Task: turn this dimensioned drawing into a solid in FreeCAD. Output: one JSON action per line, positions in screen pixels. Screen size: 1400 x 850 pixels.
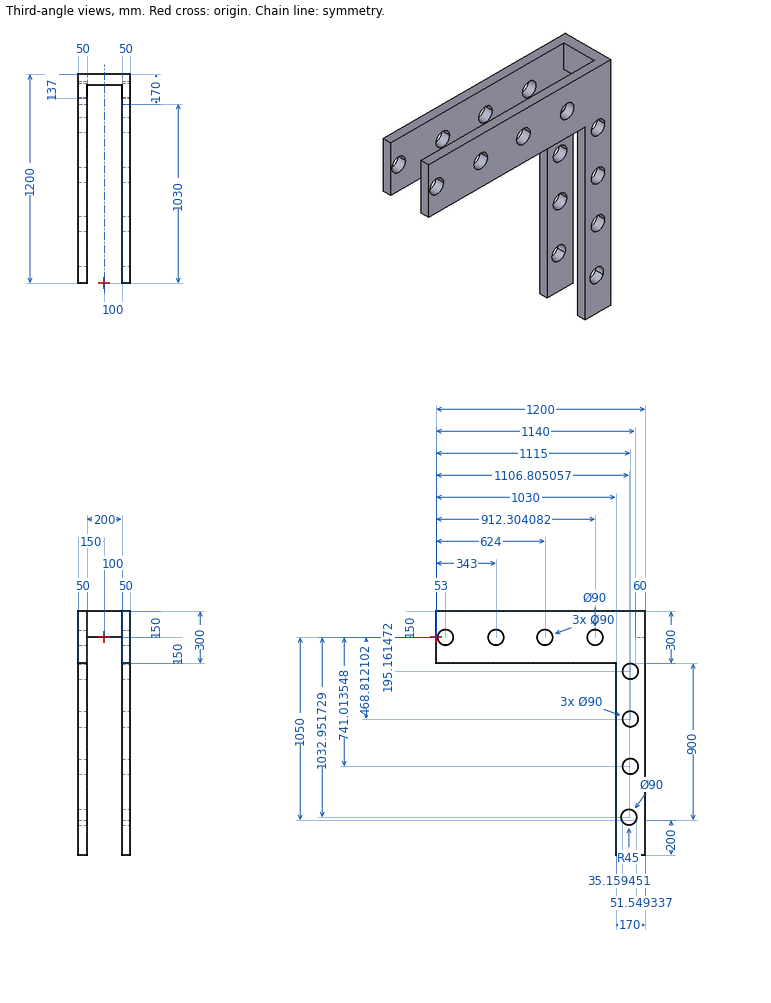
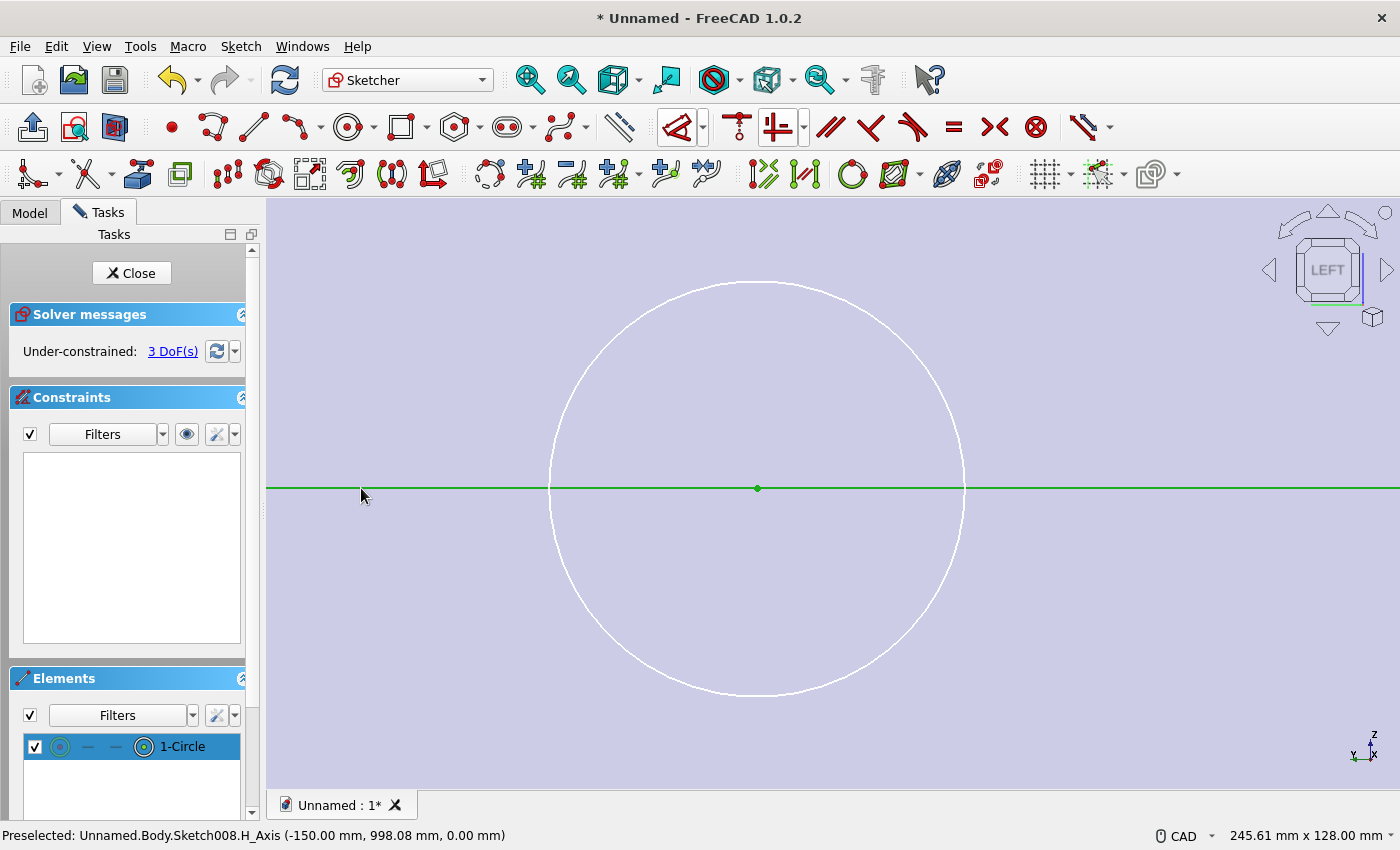
{"action": "left_click", "coordinate": [737, 128]}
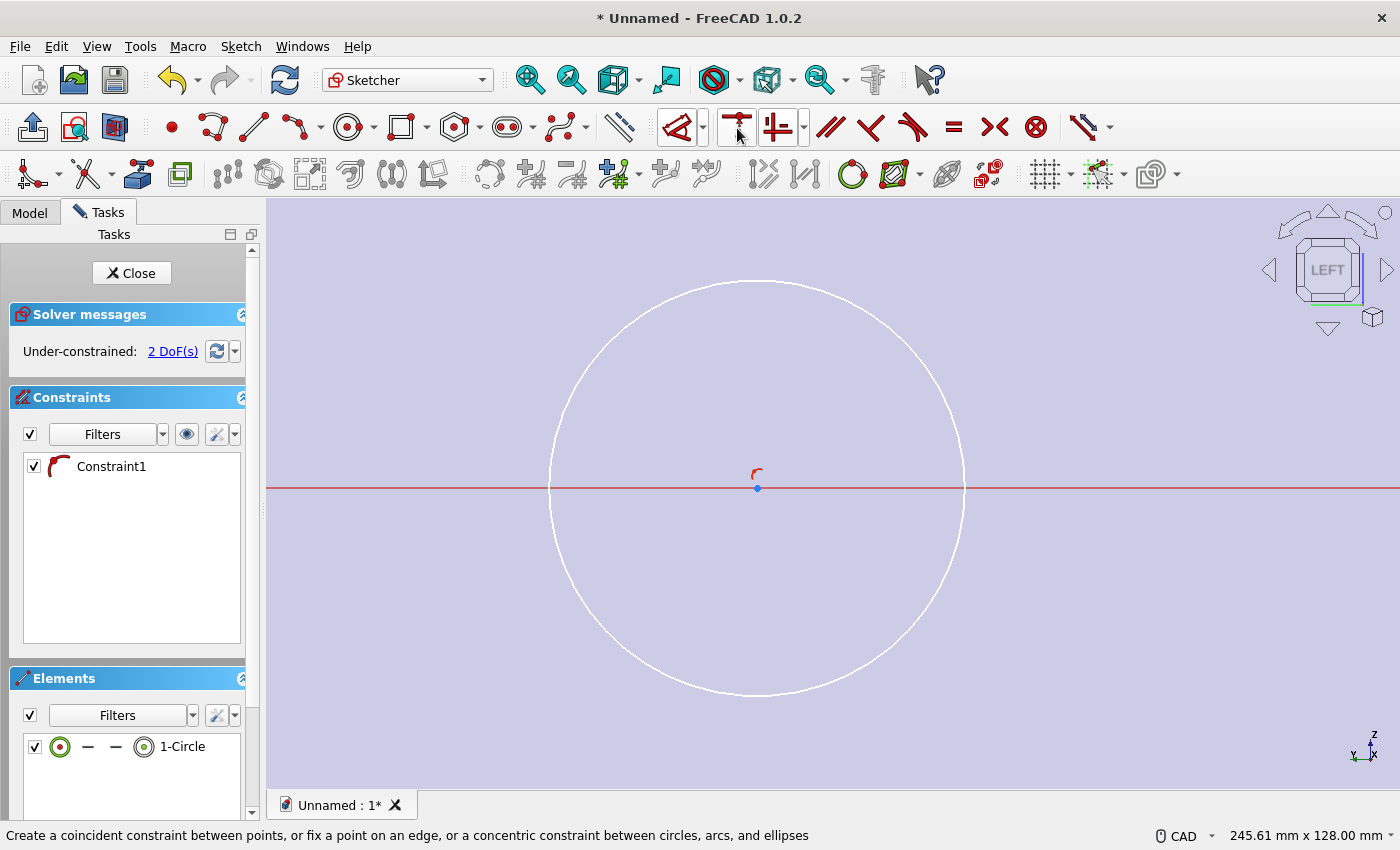
{"action": "left_click", "coordinate": [904, 341]}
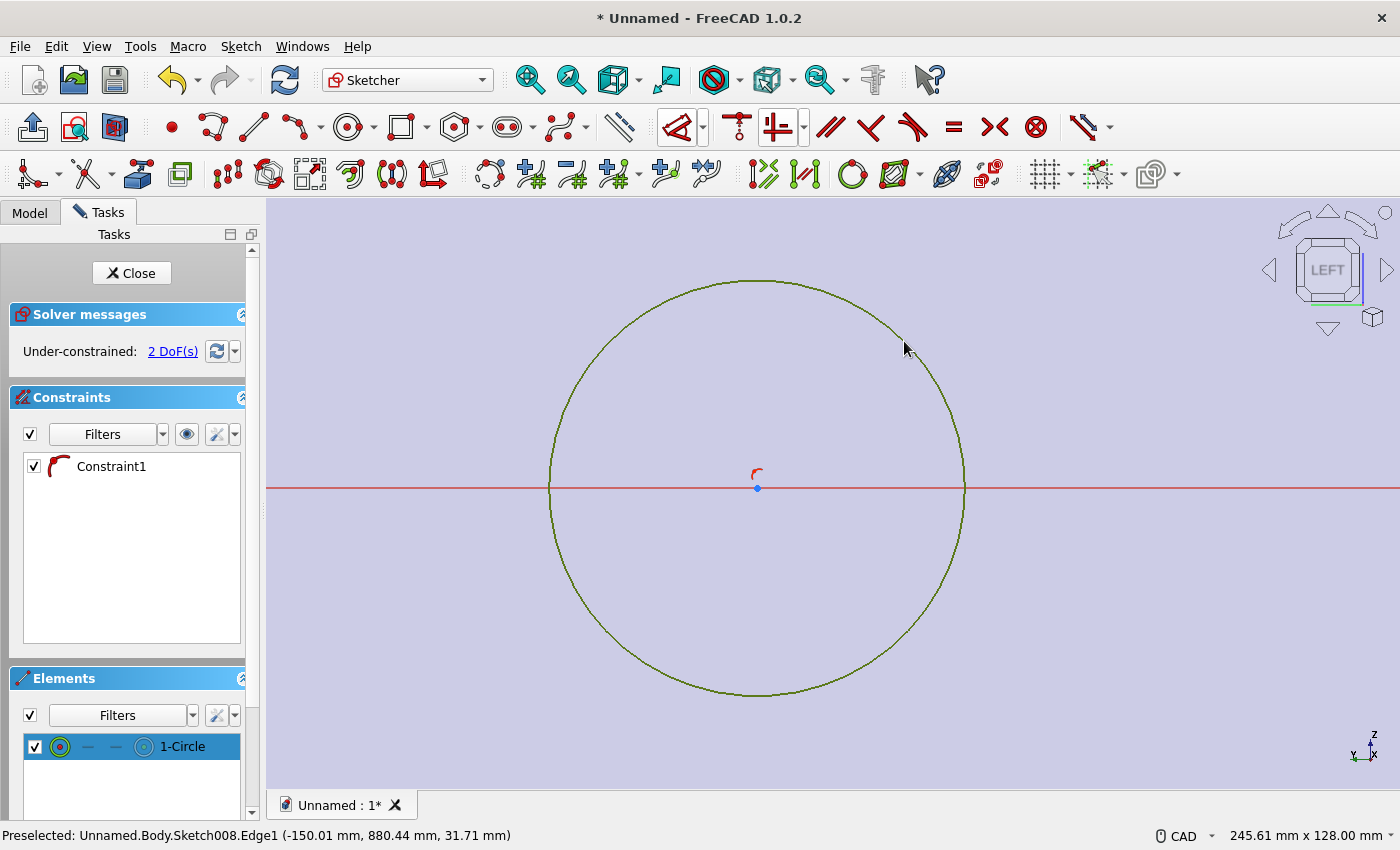
{"action": "key", "text": "k o"}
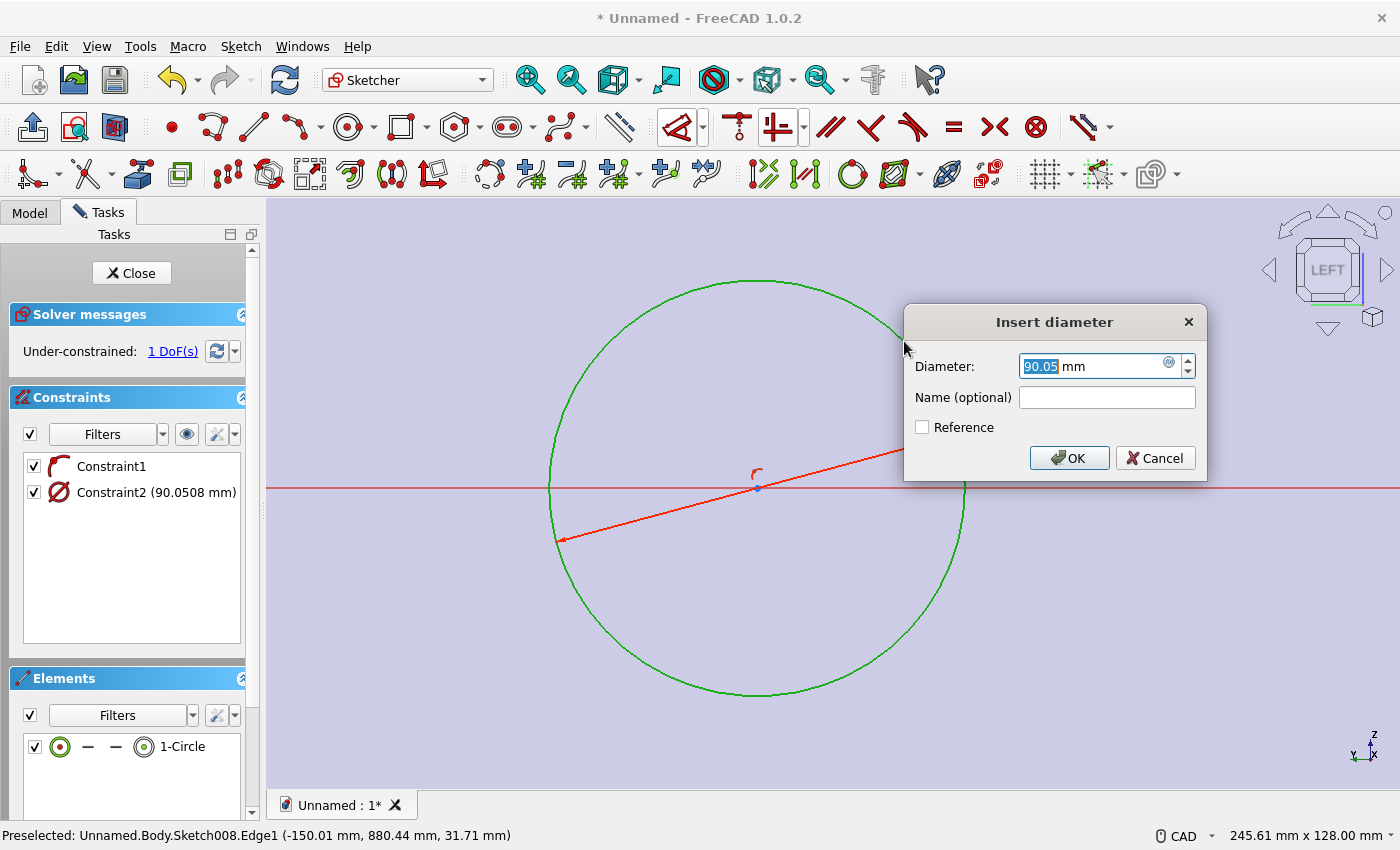
{"action": "type", "text": "90"}
{"action": "key", "text": "Return"}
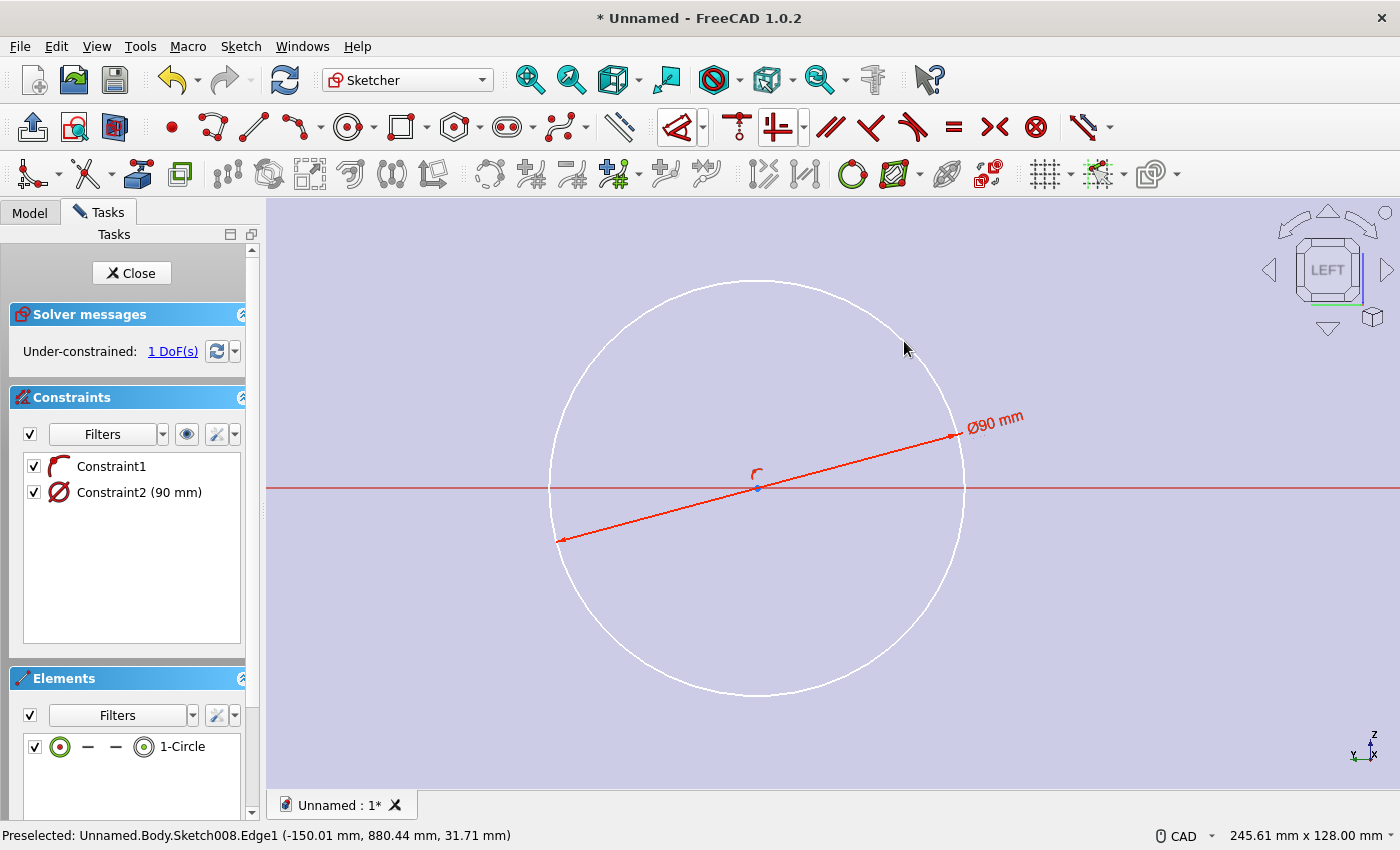
{"action": "left_click", "coordinate": [757, 488]}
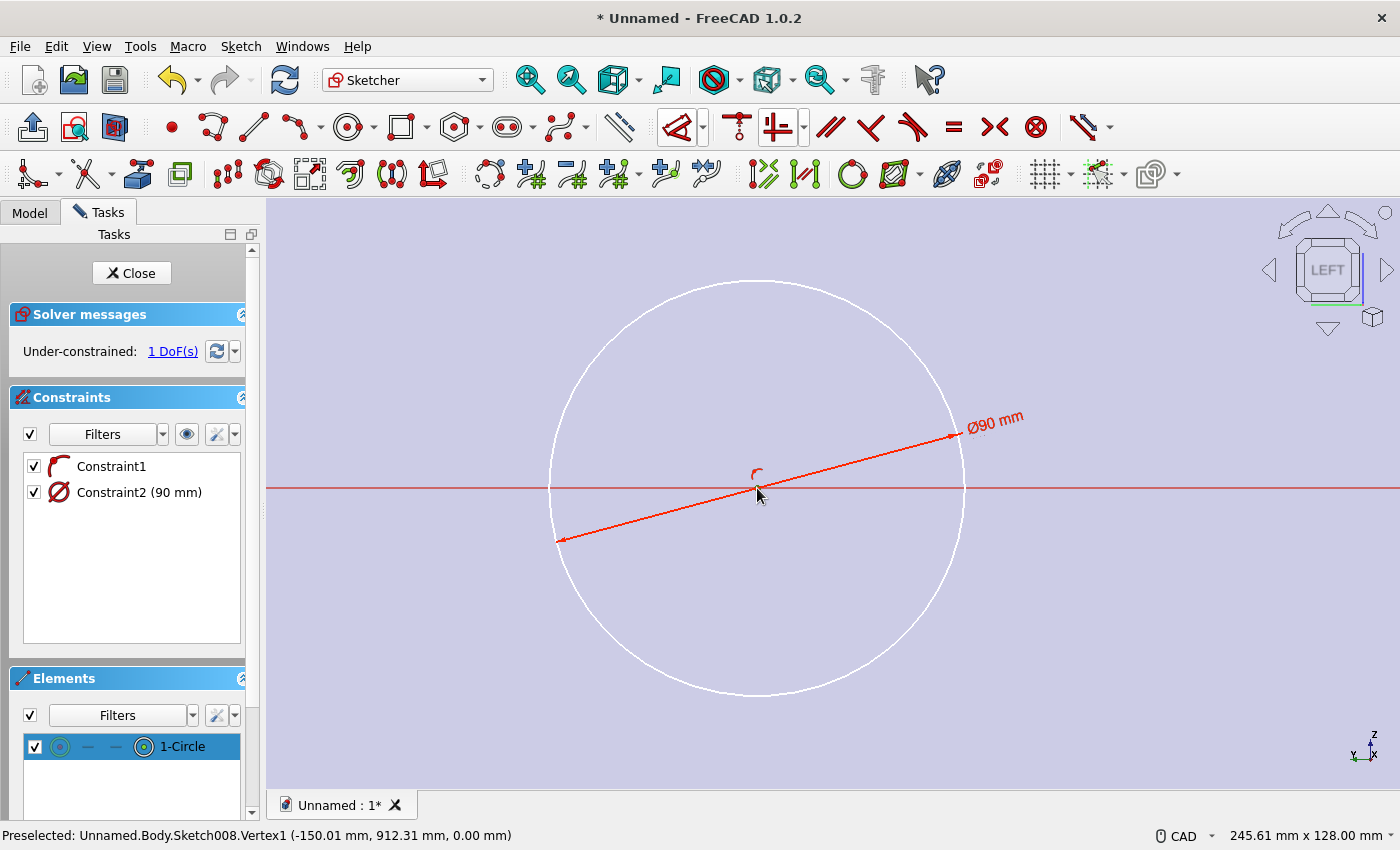
{"action": "key", "text": "l"}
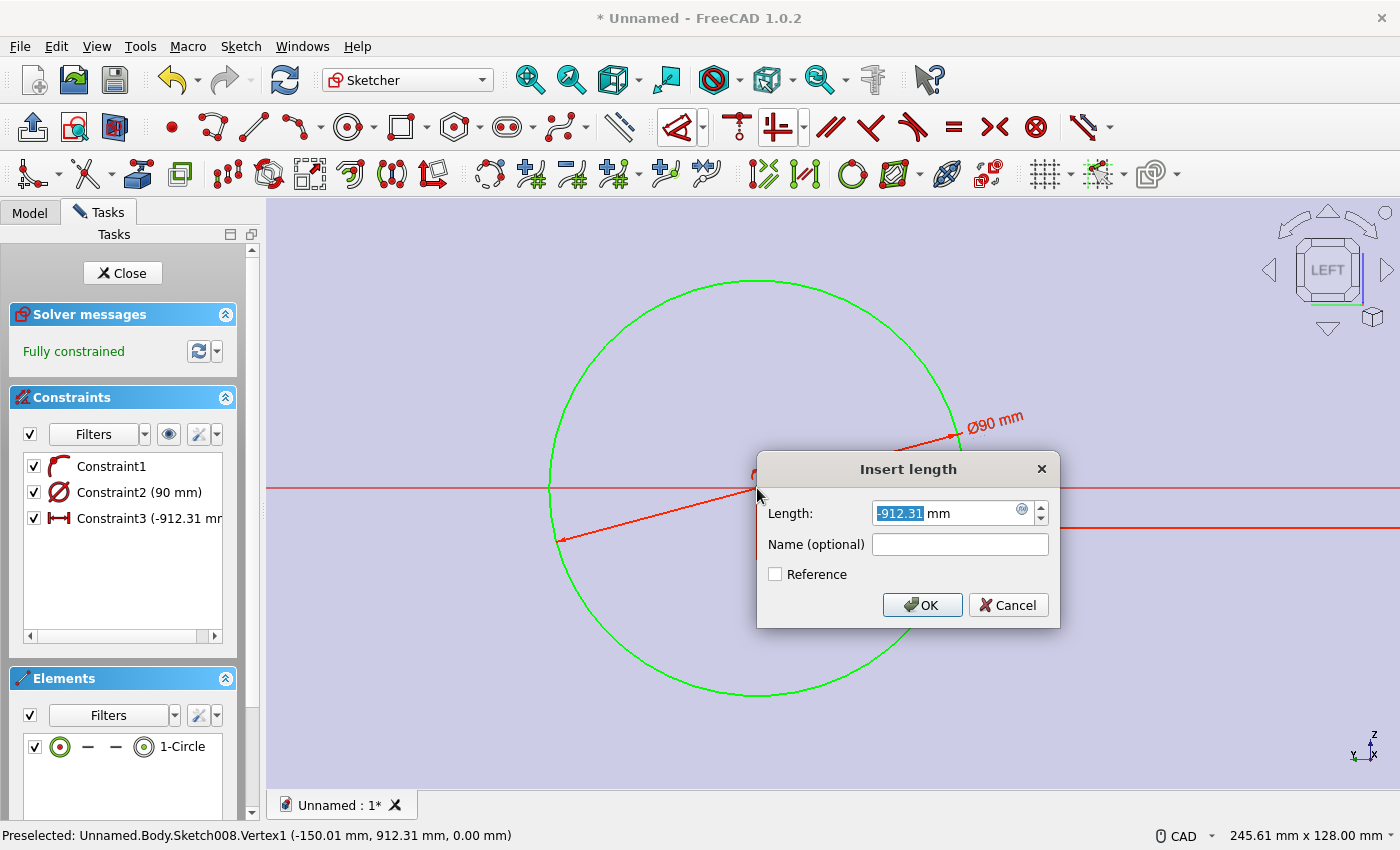
{"action": "type", "text": "-912.304082"}
{"action": "key", "text": "Return"}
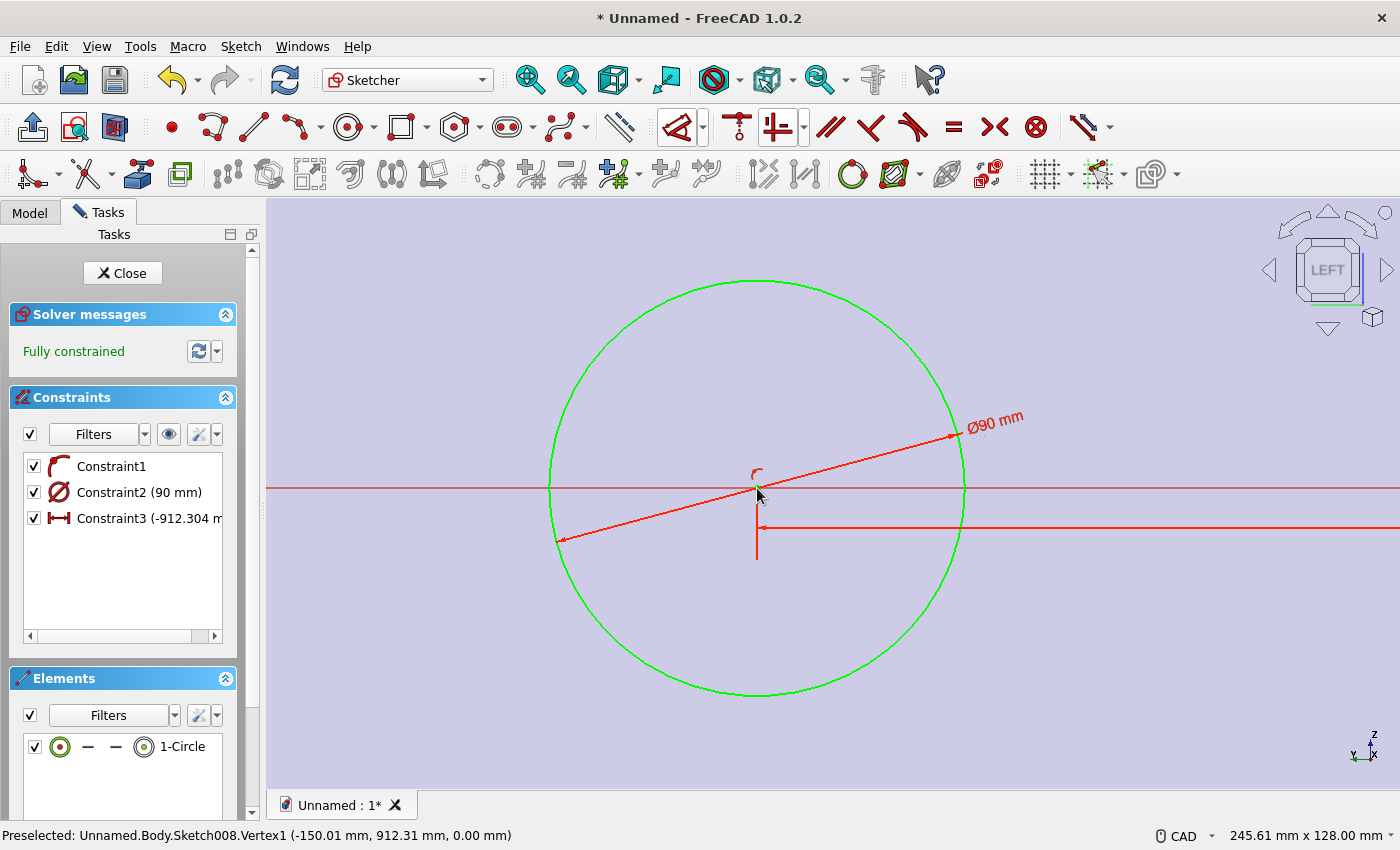
{"action": "left_click", "coordinate": [123, 273]}